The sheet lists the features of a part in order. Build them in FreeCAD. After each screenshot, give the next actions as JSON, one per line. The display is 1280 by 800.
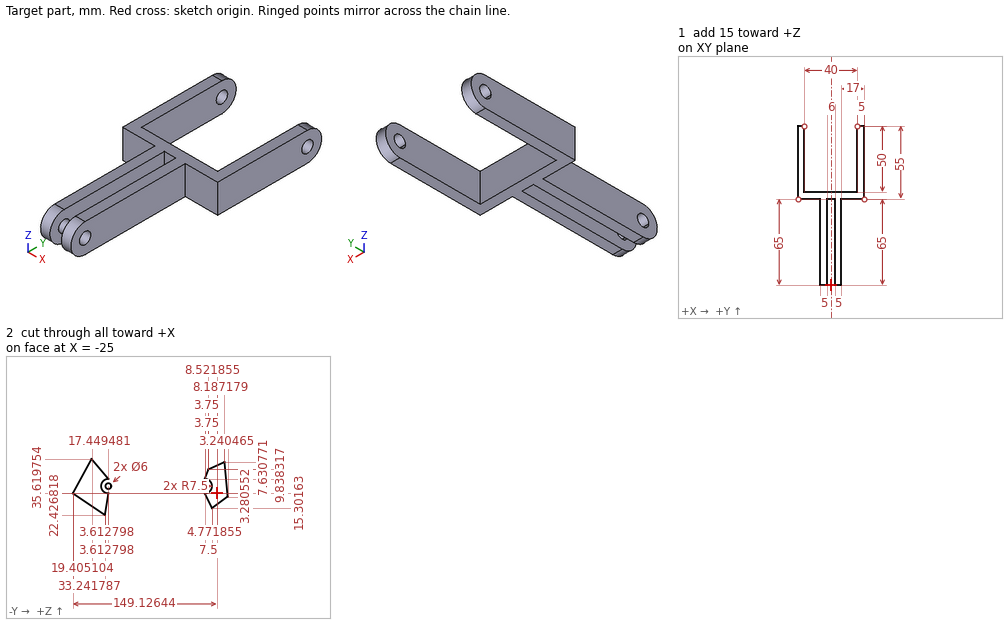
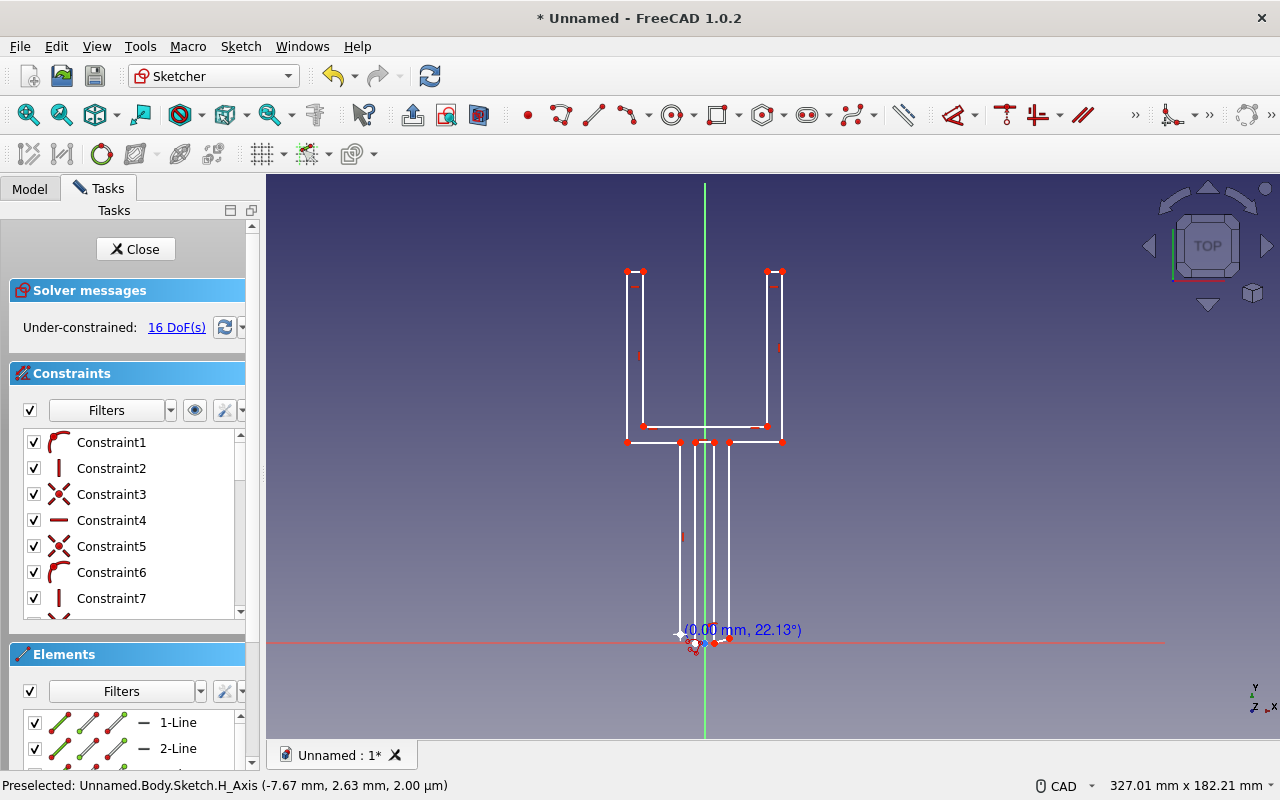
{"action": "scroll", "coordinate": [695, 643], "scroll_direction": "up", "scroll_amount": 3}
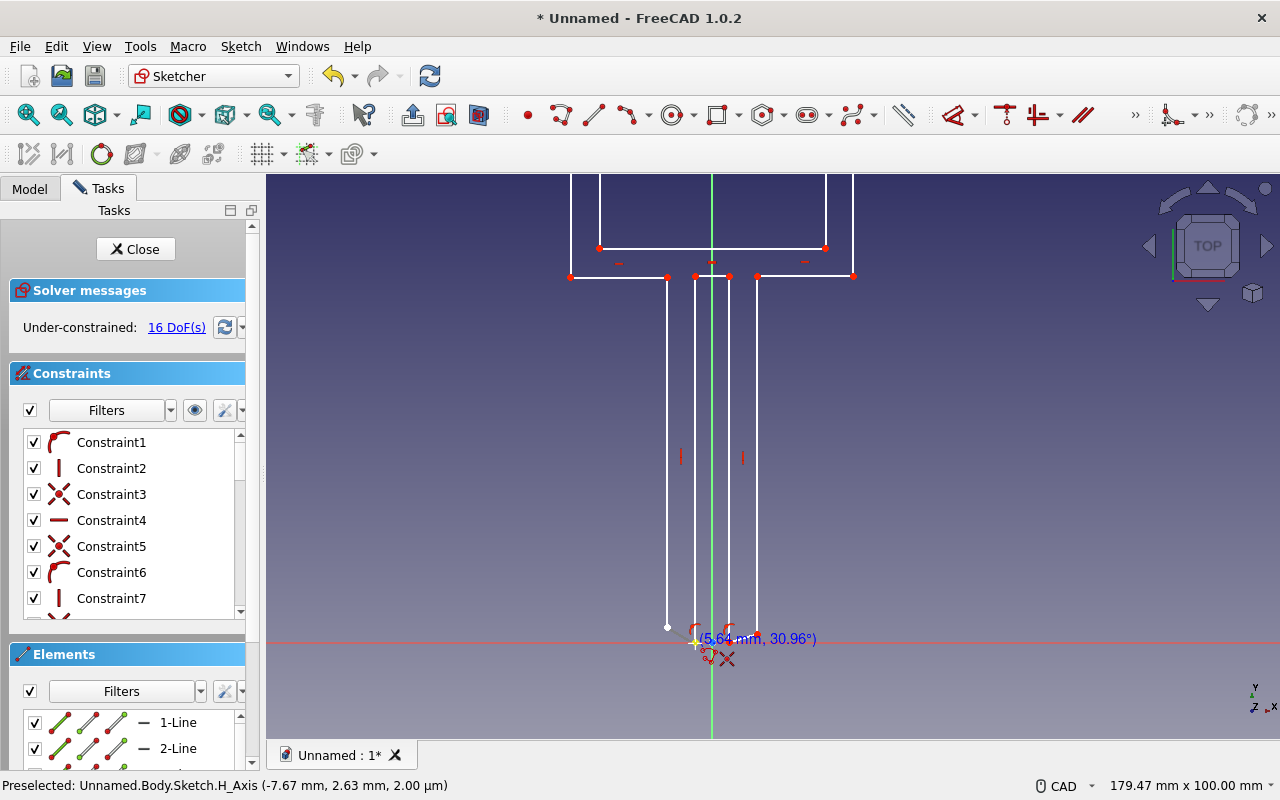
{"action": "left_click", "coordinate": [695, 643]}
{"action": "key", "text": "Escape"}
{"action": "key", "text": "Escape"}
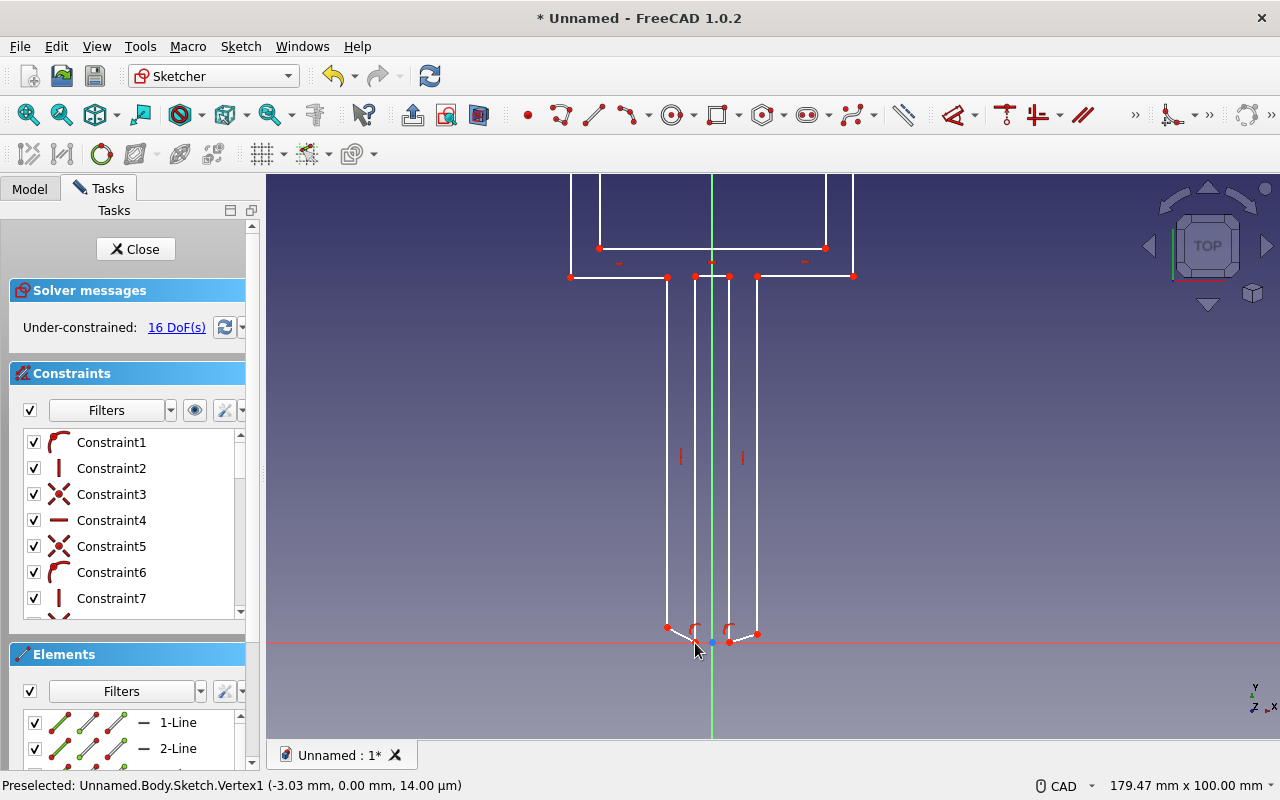
{"action": "scroll", "coordinate": [741, 639], "scroll_direction": "up", "scroll_amount": 2}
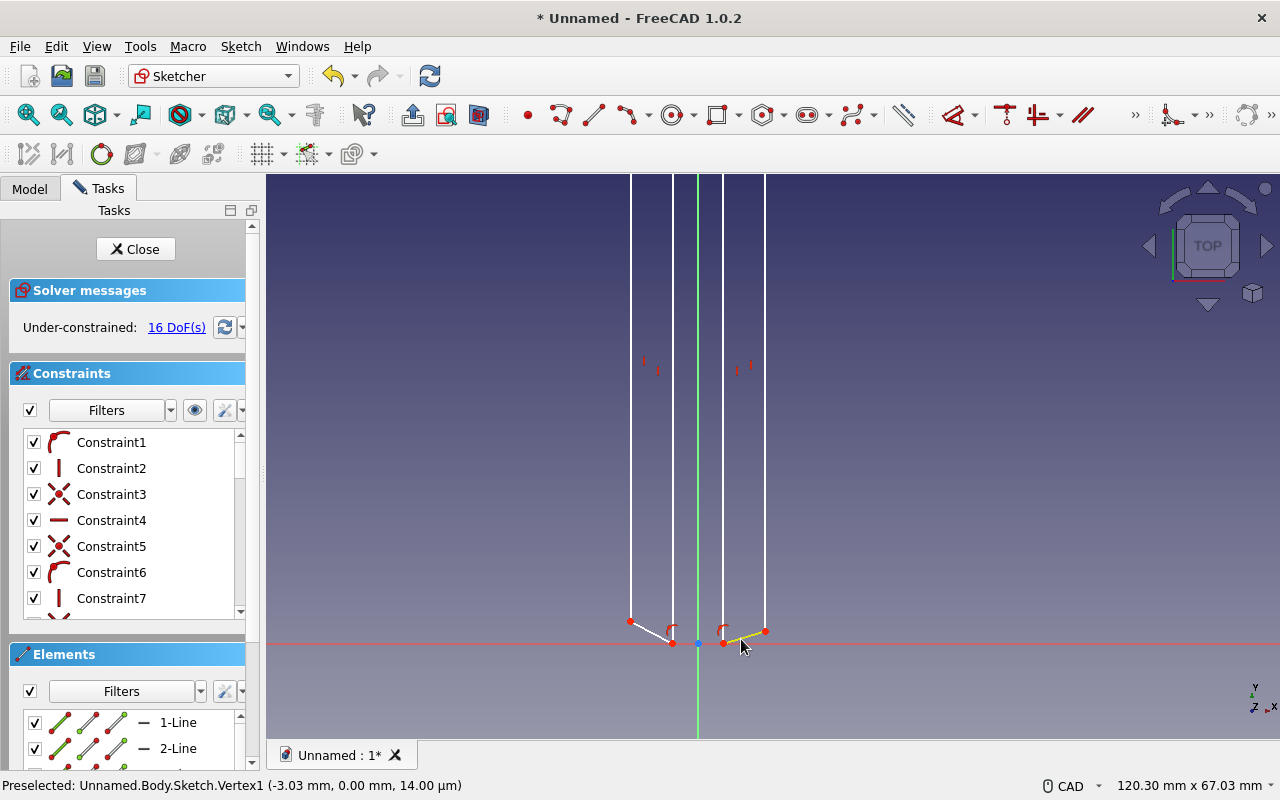
{"action": "left_click", "coordinate": [740, 639]}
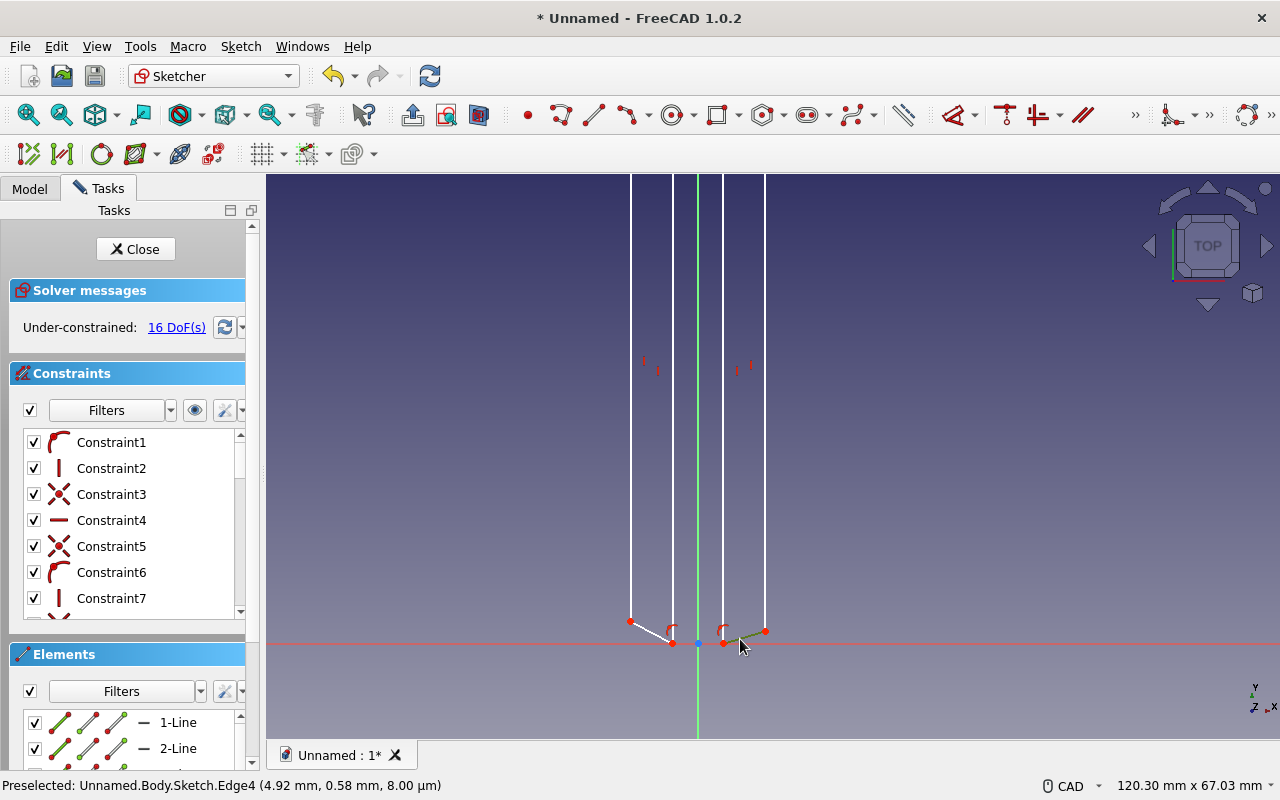
{"action": "key", "text": "h"}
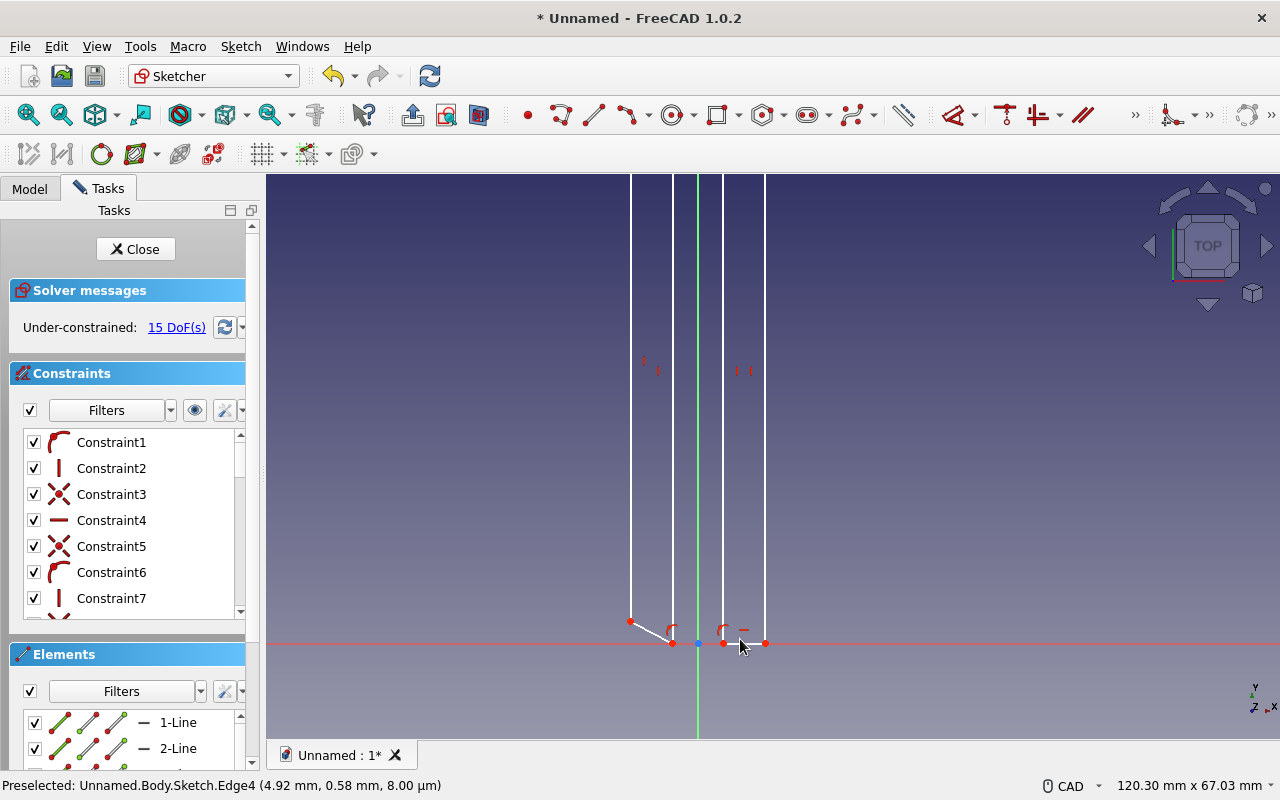
{"action": "left_click", "coordinate": [643, 628]}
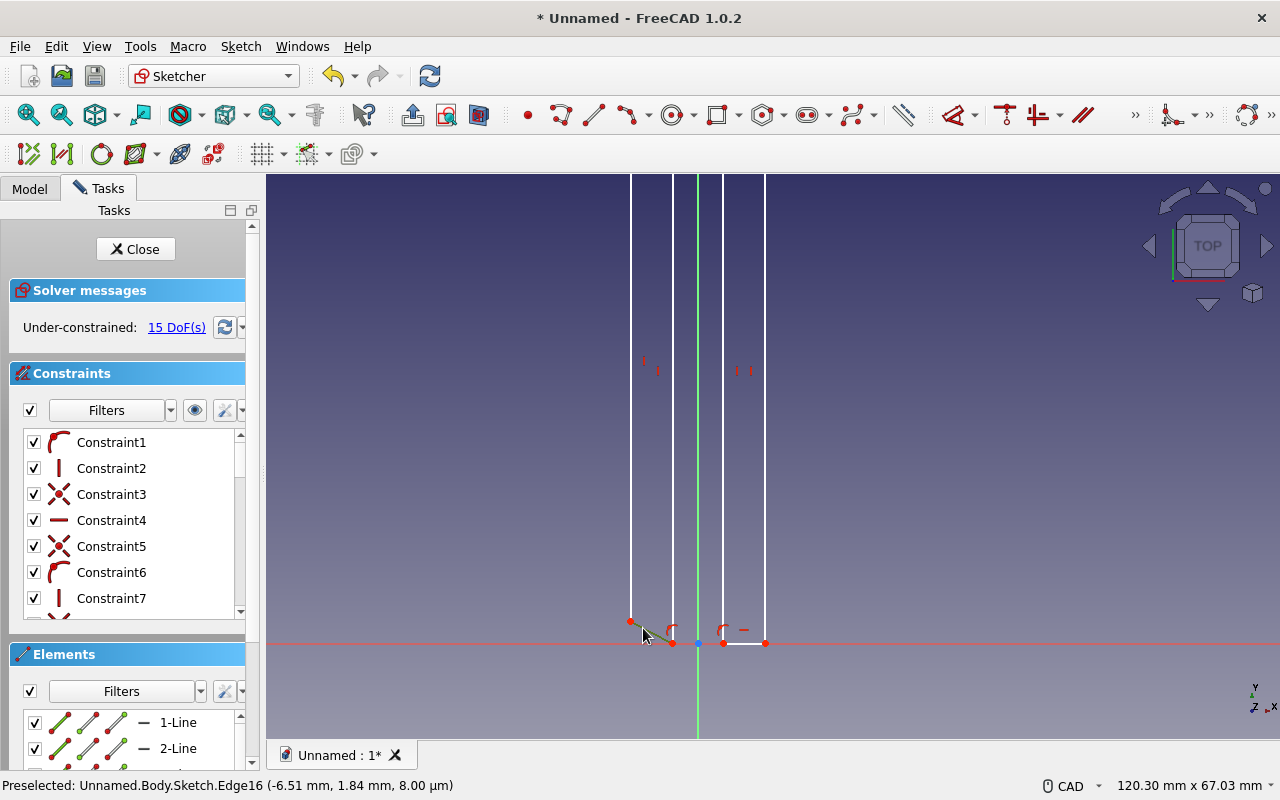
{"action": "key", "text": "h"}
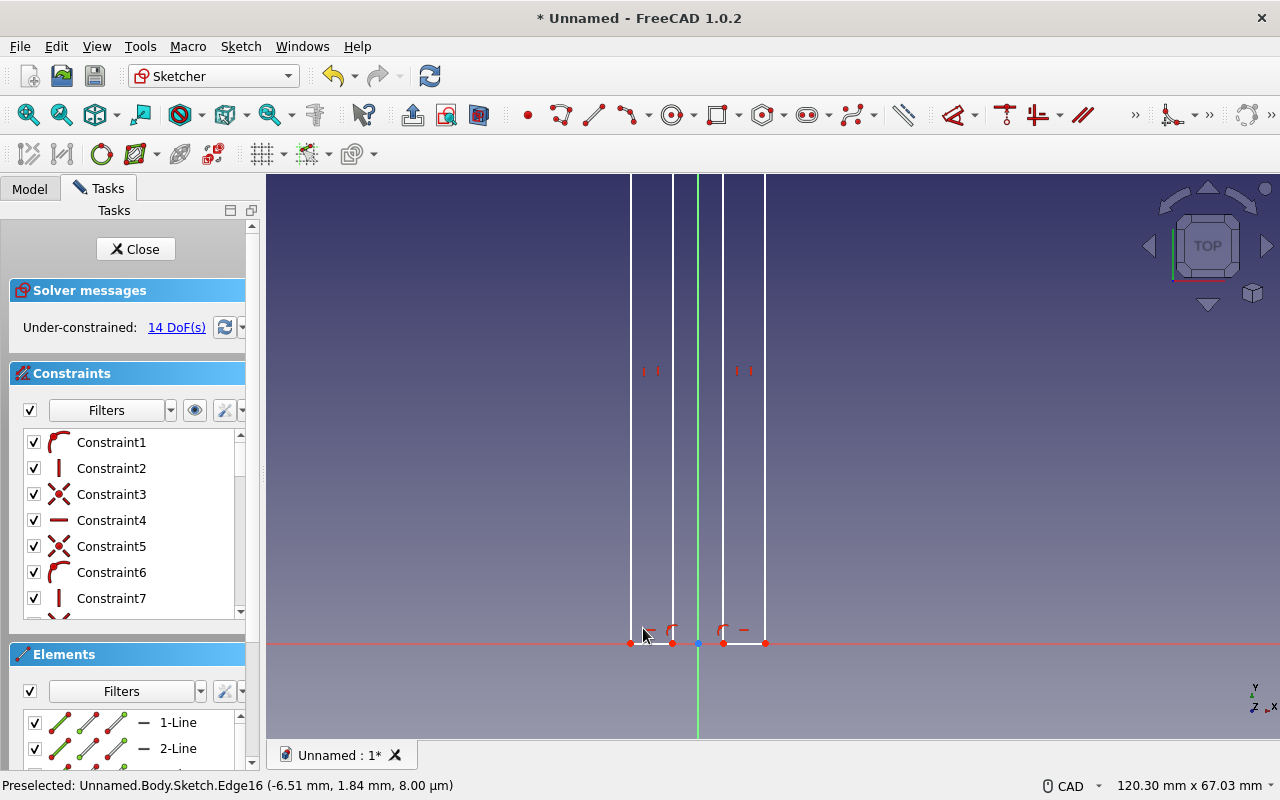
{"action": "scroll", "coordinate": [708, 642], "scroll_direction": "down", "scroll_amount": 5}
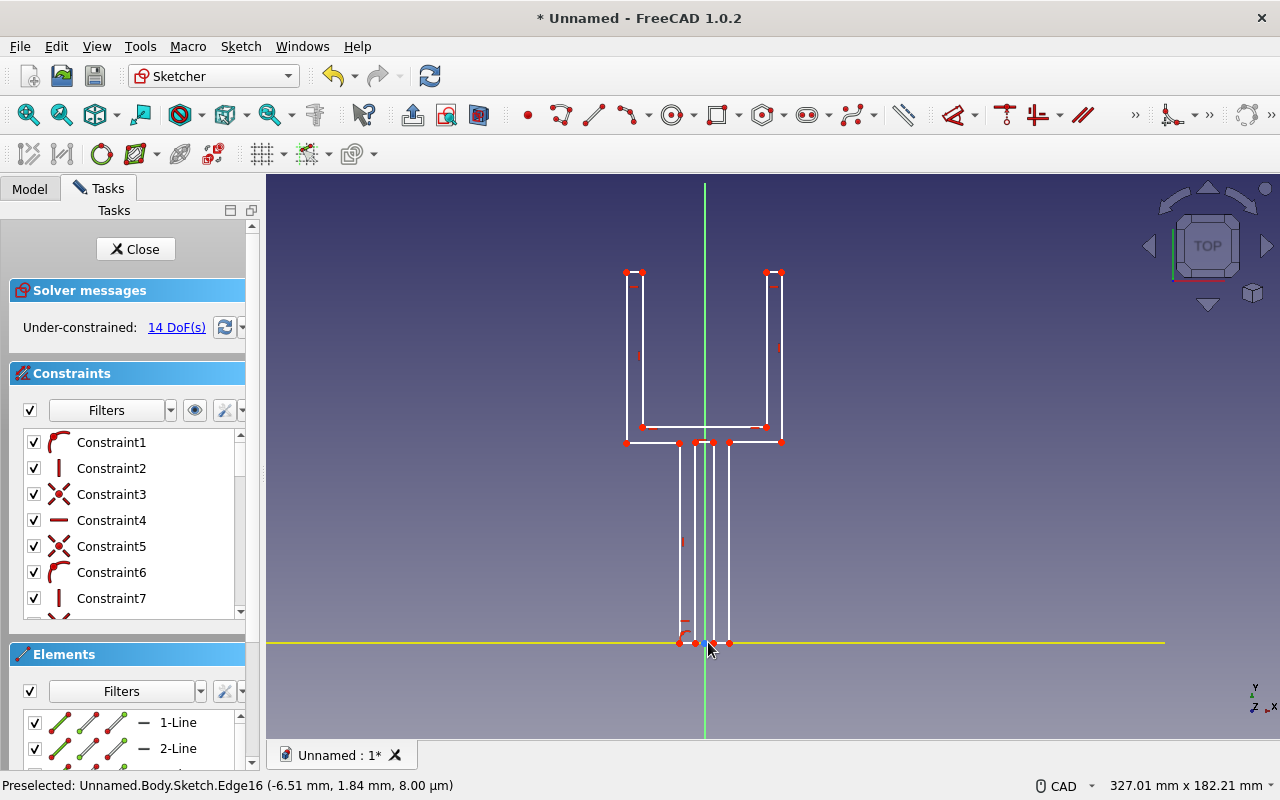
{"action": "left_click", "coordinate": [767, 272]}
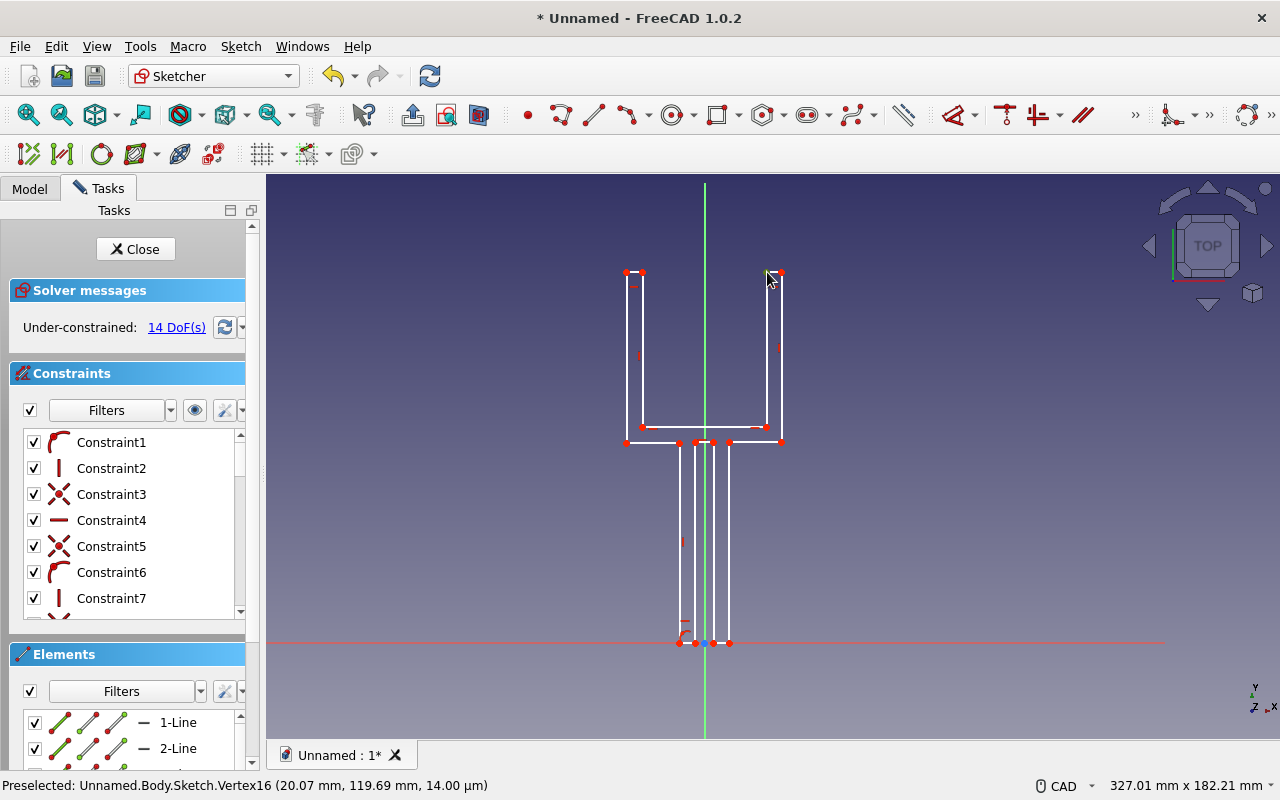
{"action": "left_click", "coordinate": [643, 272]}